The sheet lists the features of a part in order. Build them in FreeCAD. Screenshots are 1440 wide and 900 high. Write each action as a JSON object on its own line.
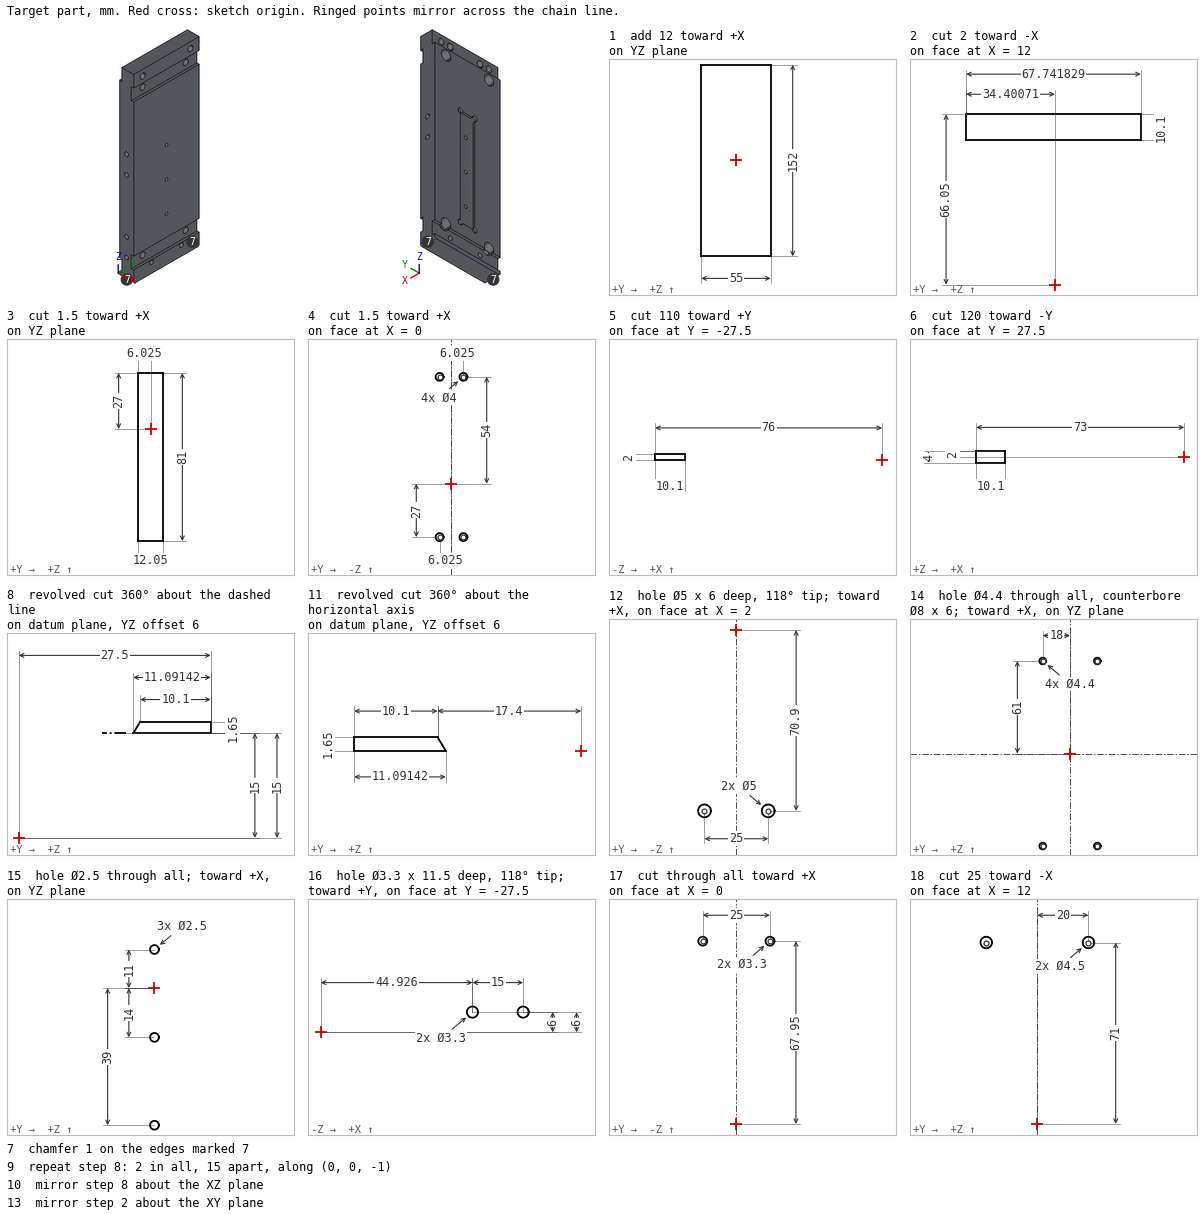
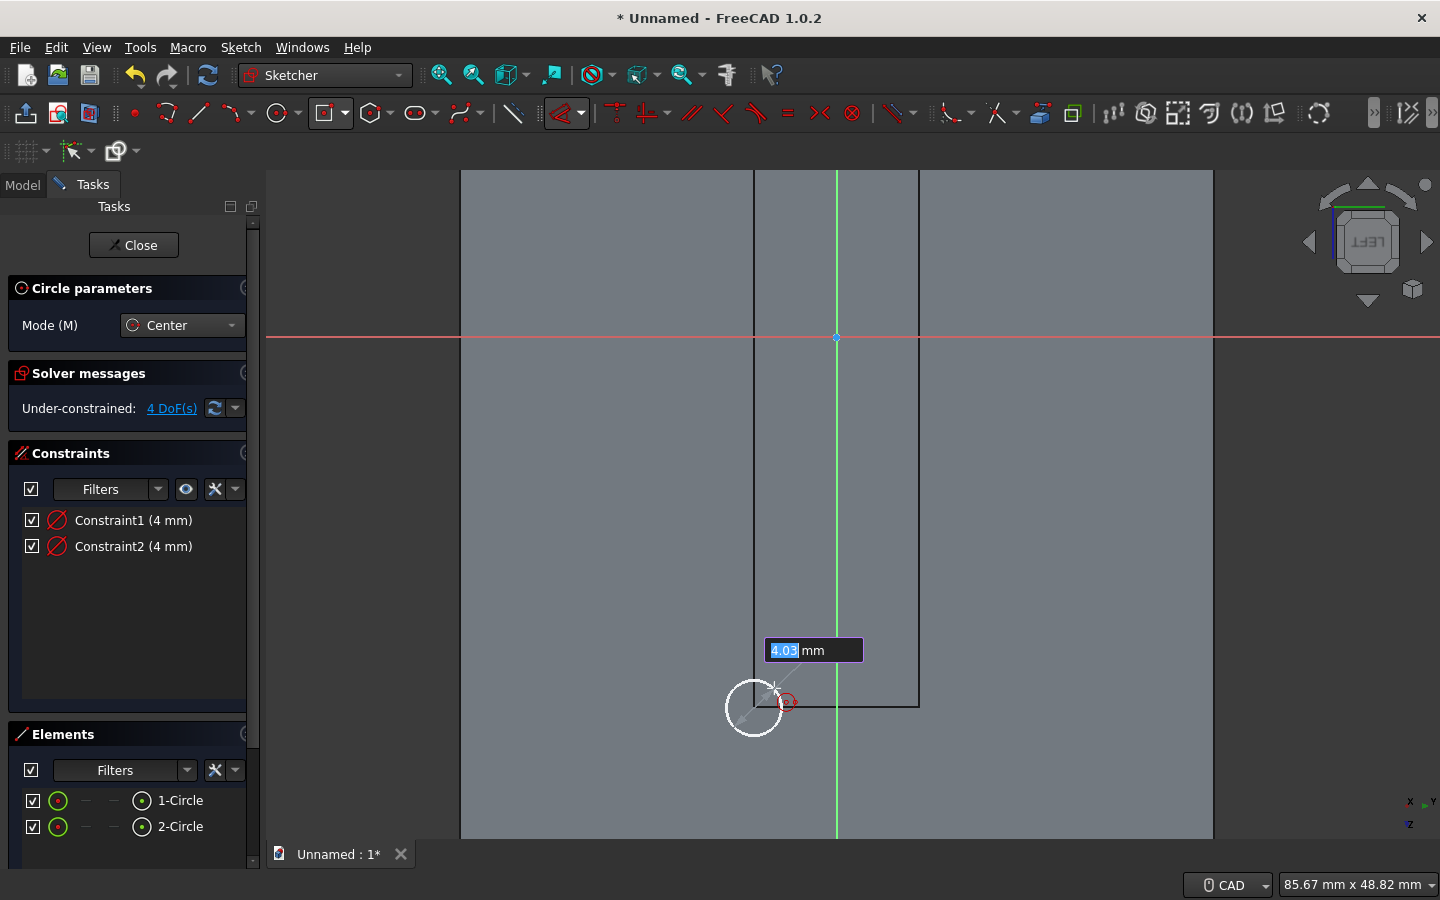
{"action": "type", "text": "4"}
{"action": "key", "text": "Return"}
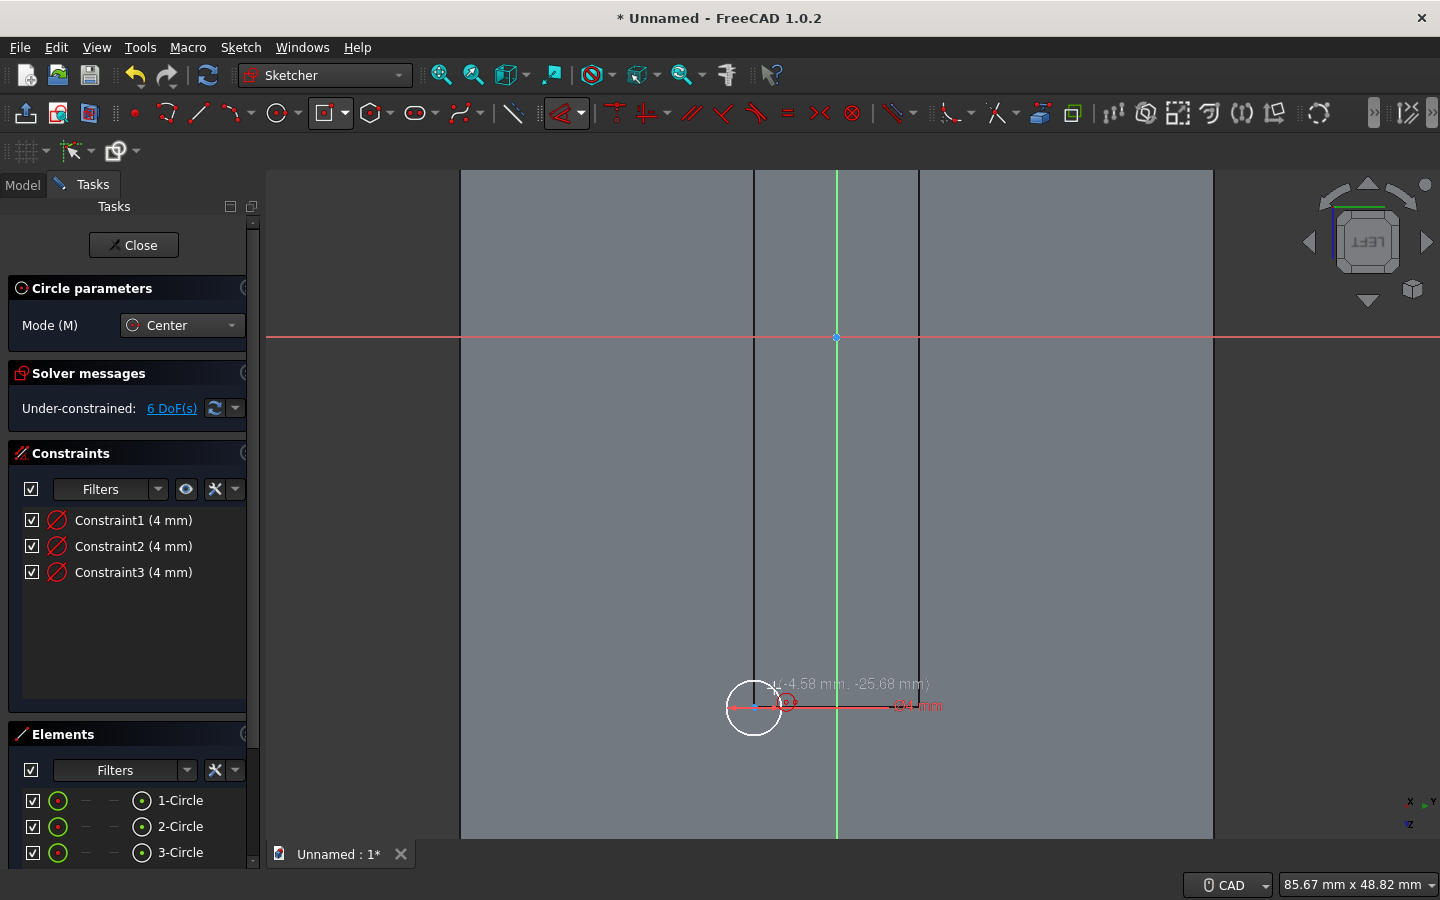
{"action": "left_click", "coordinate": [919, 707]}
{"action": "mouse_move", "coordinate": [939, 688]}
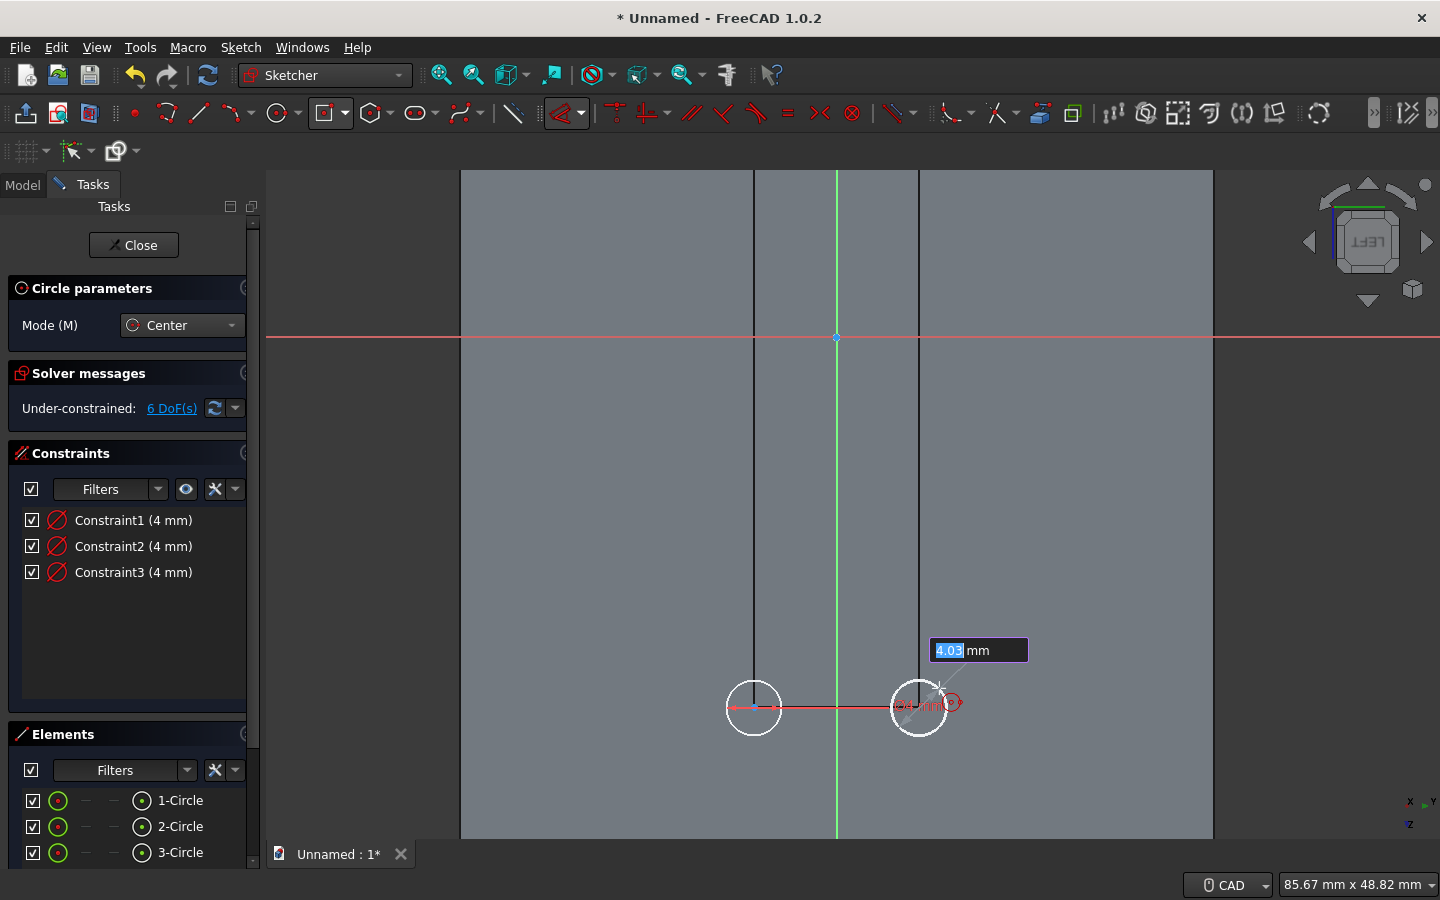
{"action": "type", "text": "4"}
{"action": "key", "text": "Return"}
{"action": "key", "text": "Escape"}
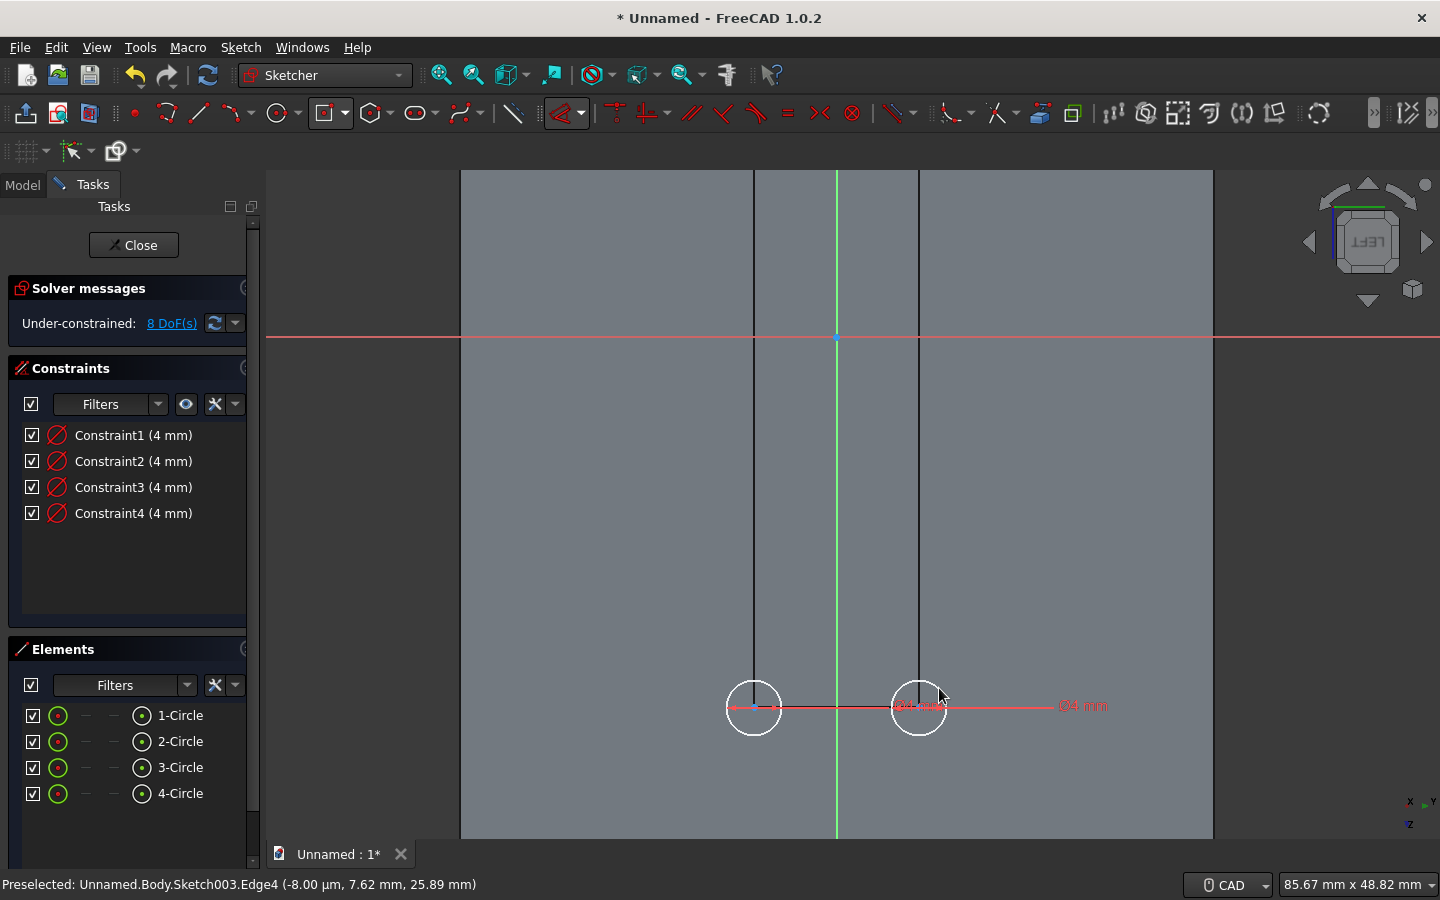
{"action": "scroll", "coordinate": [754, 710], "scroll_direction": "down", "scroll_amount": 5}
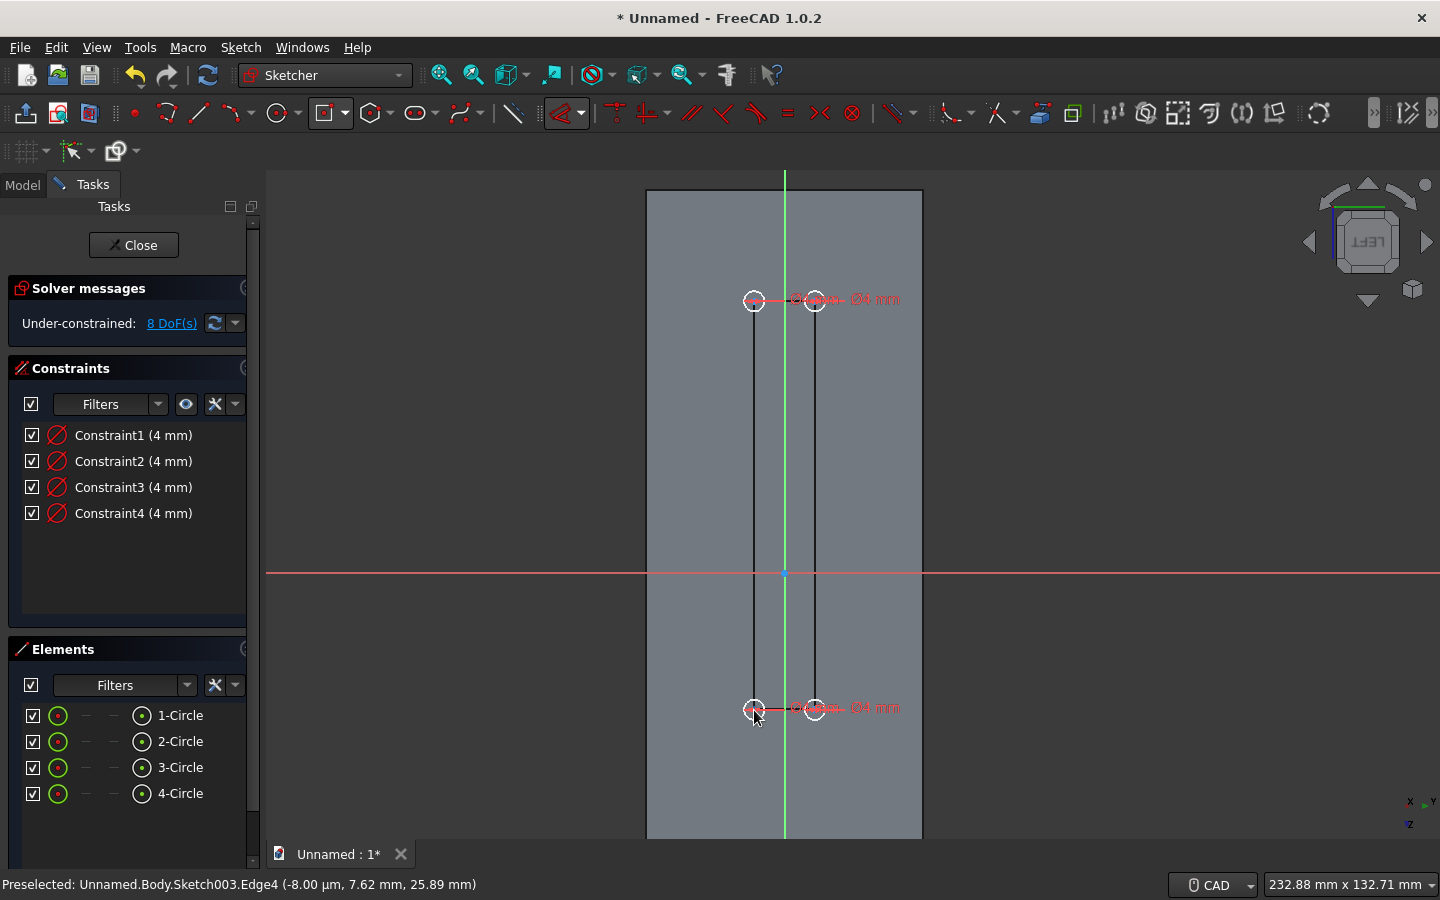
{"action": "left_click", "coordinate": [815, 301]}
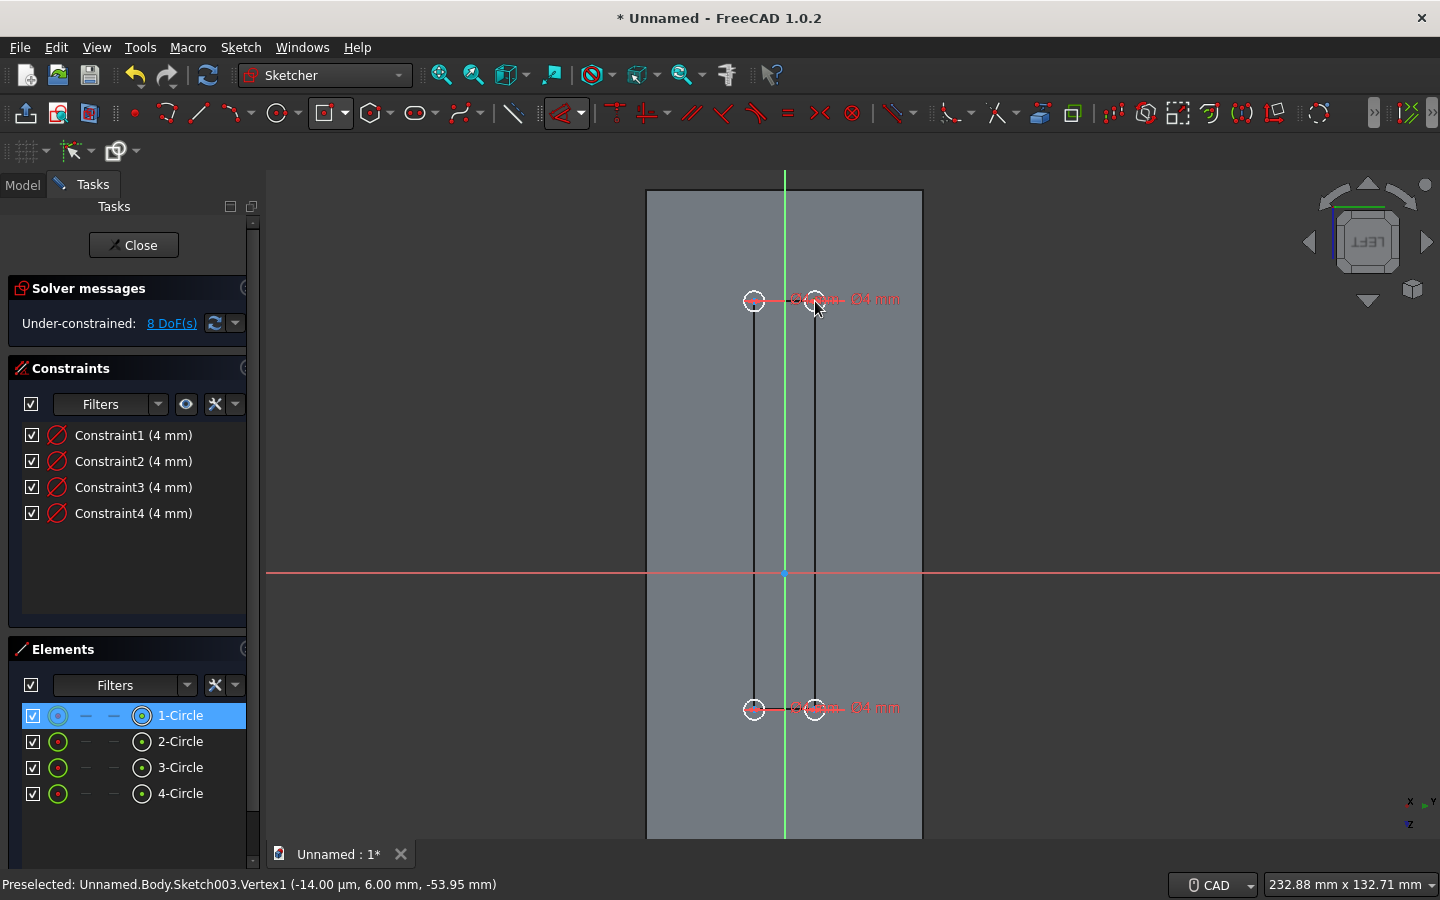
{"action": "left_click", "coordinate": [754, 301]}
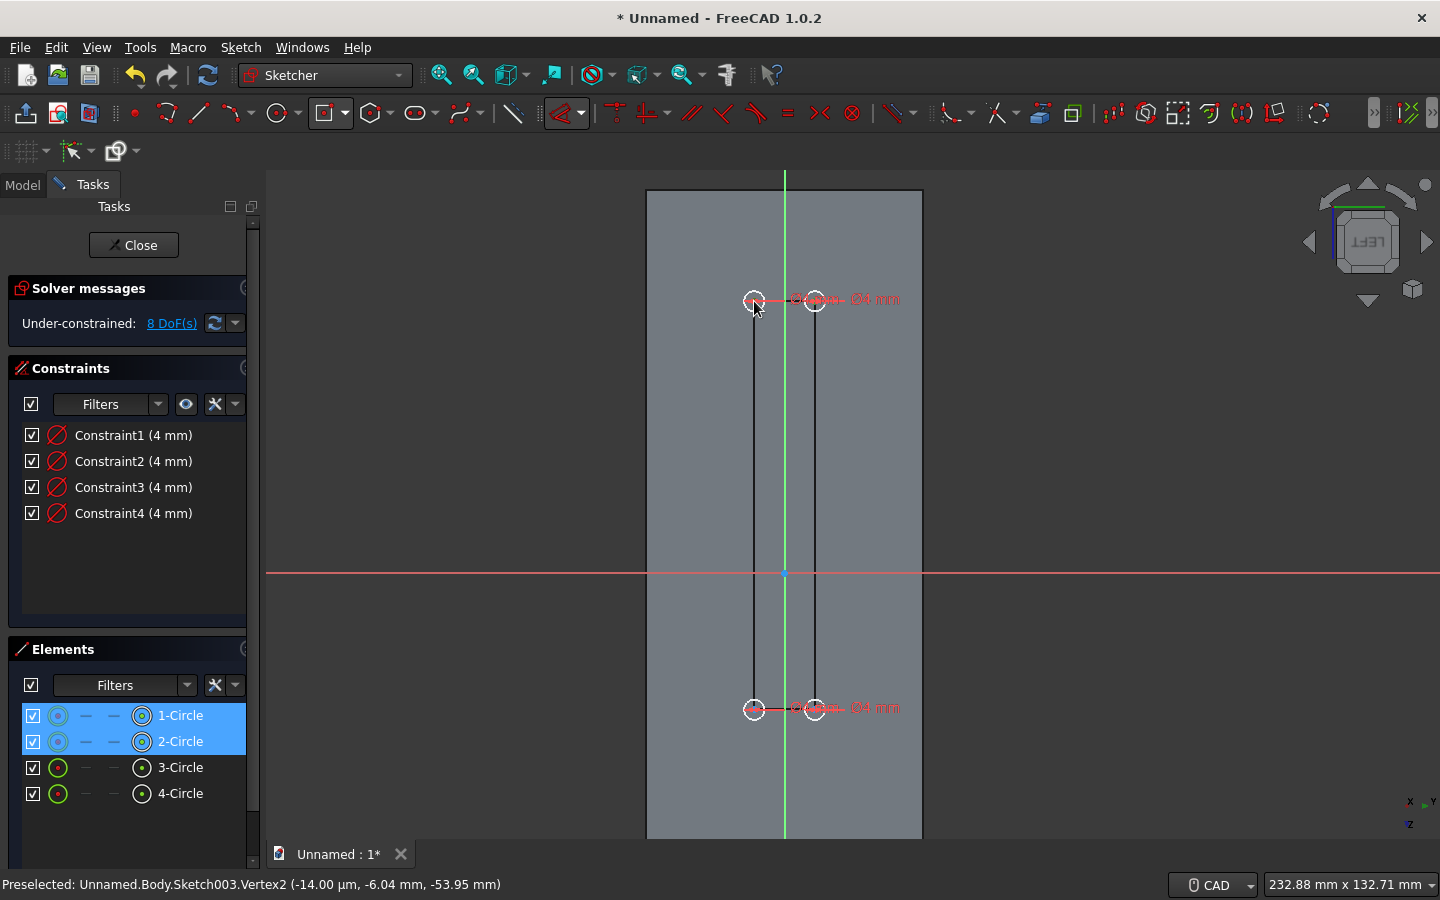
{"action": "left_click", "coordinate": [785, 767]}